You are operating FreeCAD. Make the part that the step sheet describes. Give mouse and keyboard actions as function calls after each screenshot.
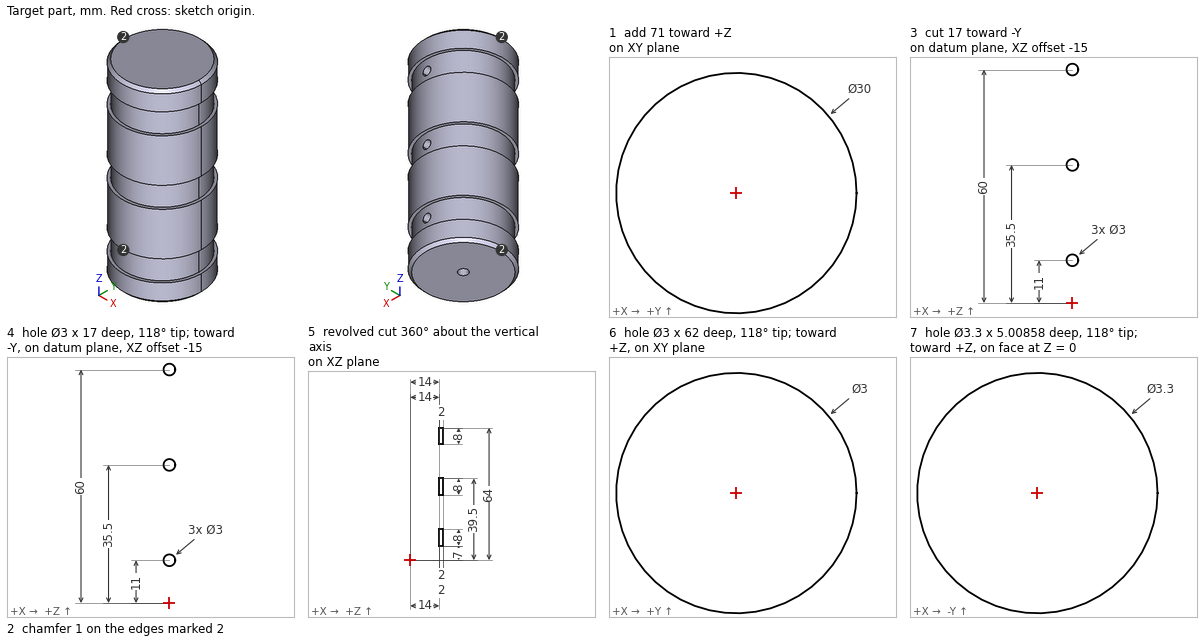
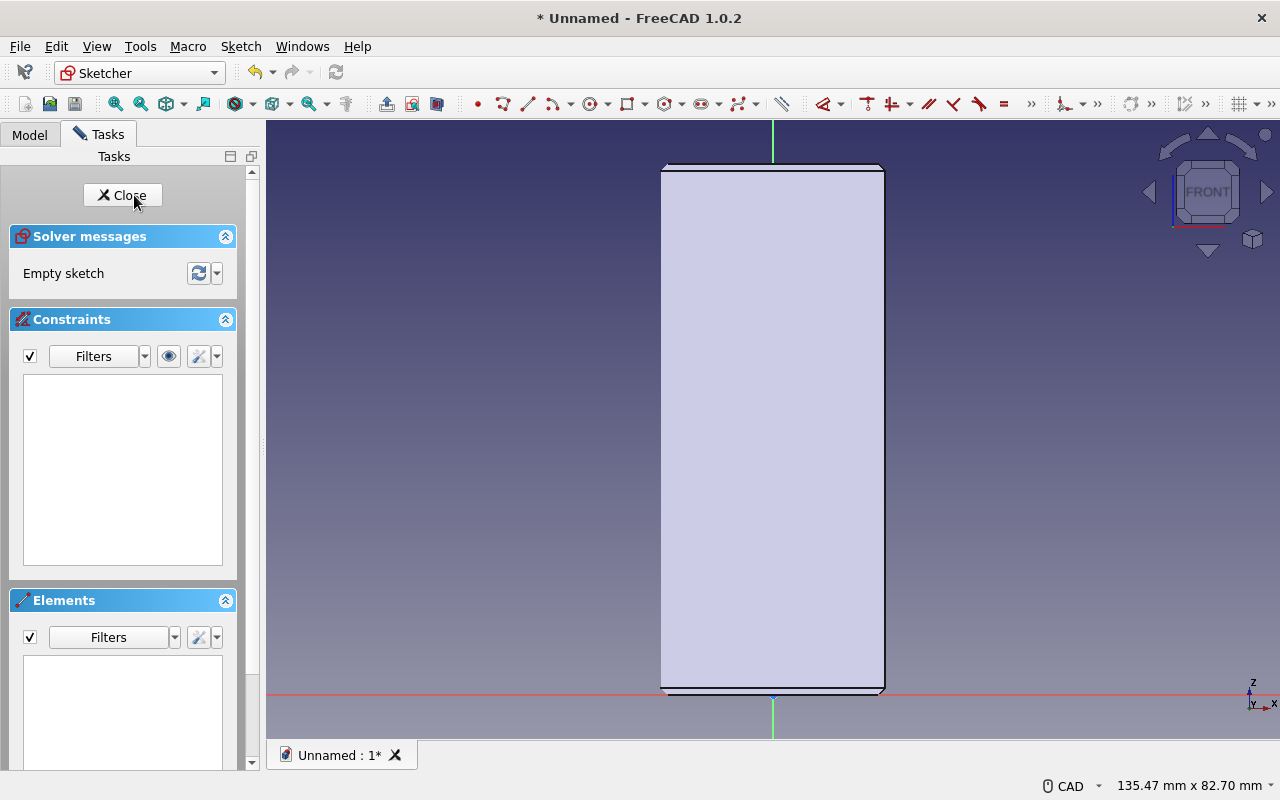
click(437, 104)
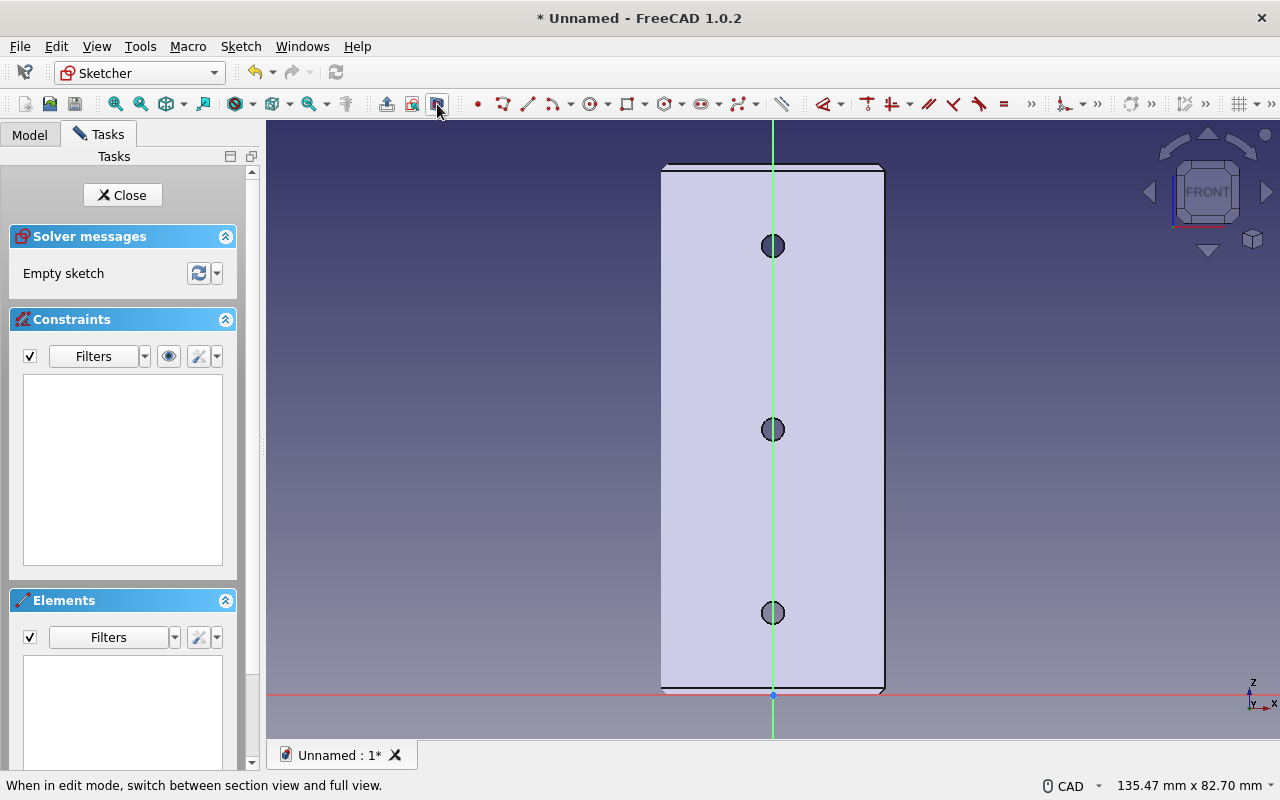
scroll(294, 311, down, 1)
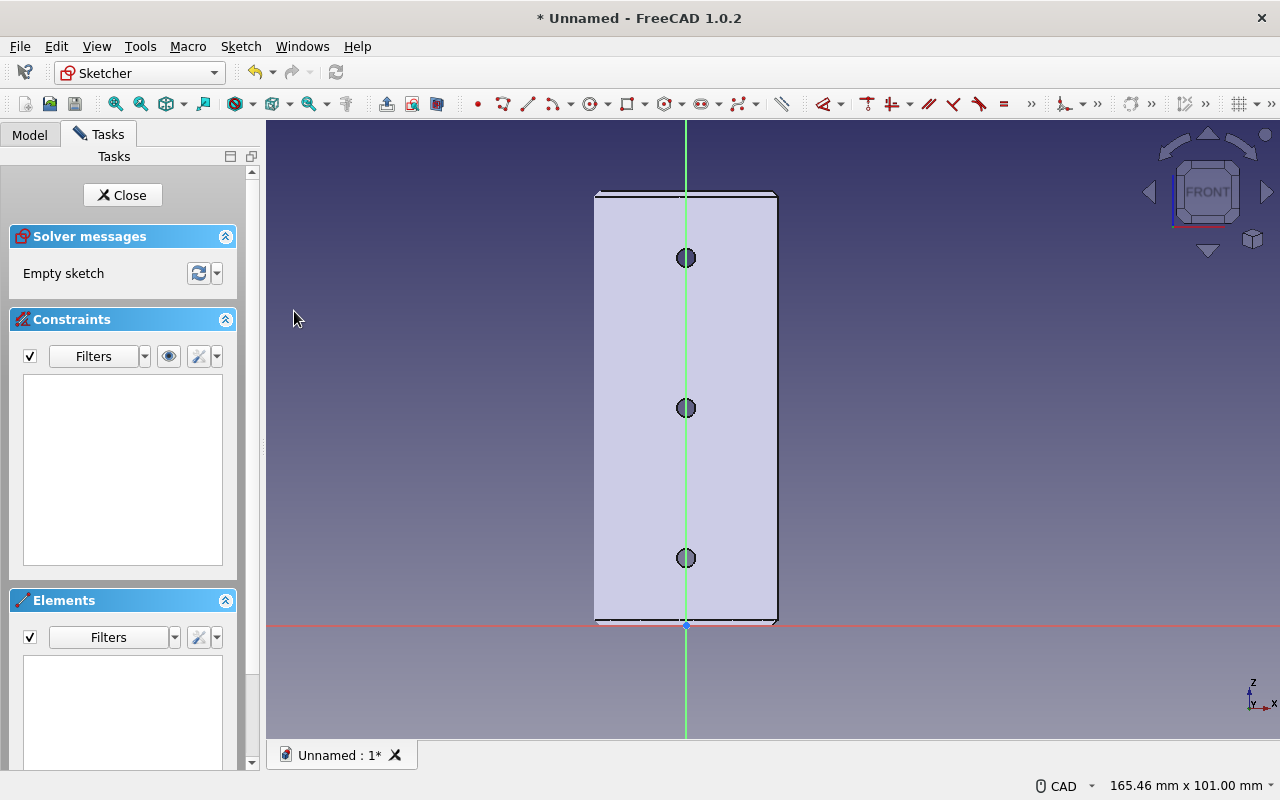
click(626, 104)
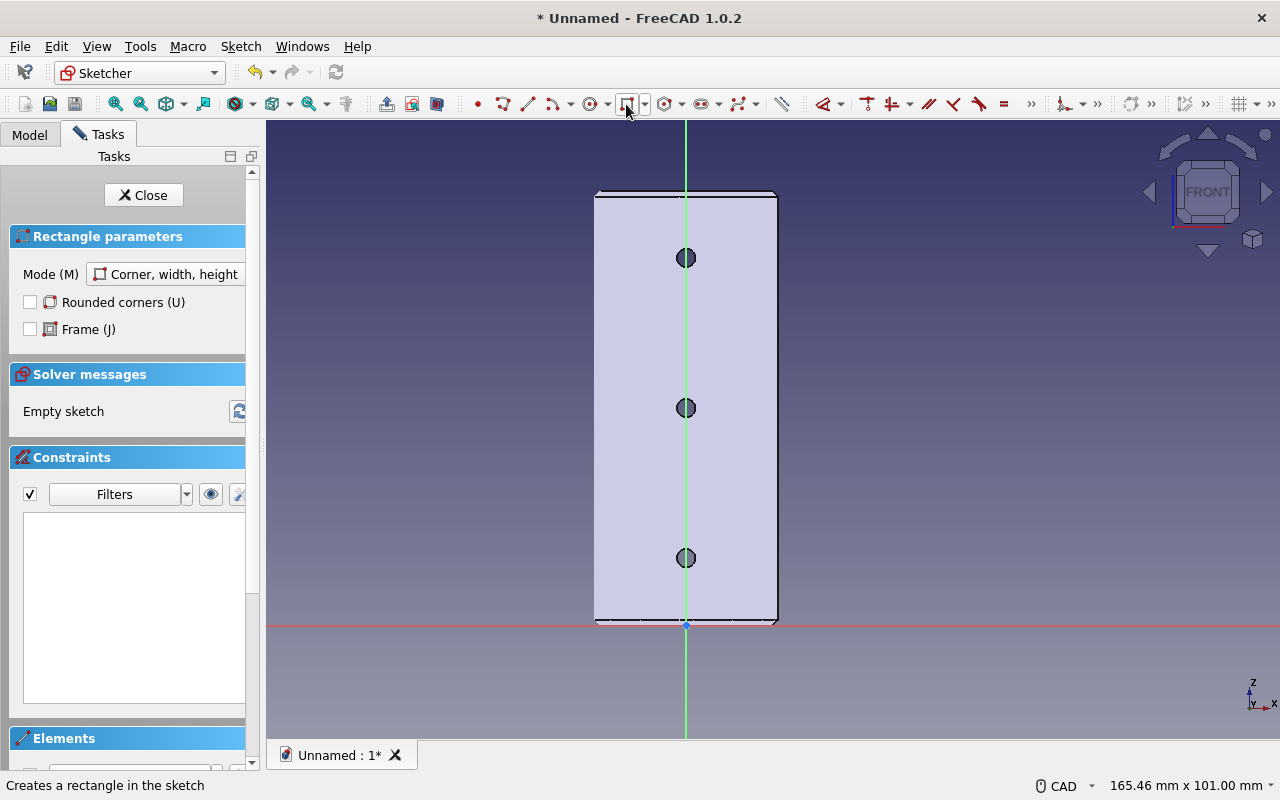
scroll(772, 534, up, 2)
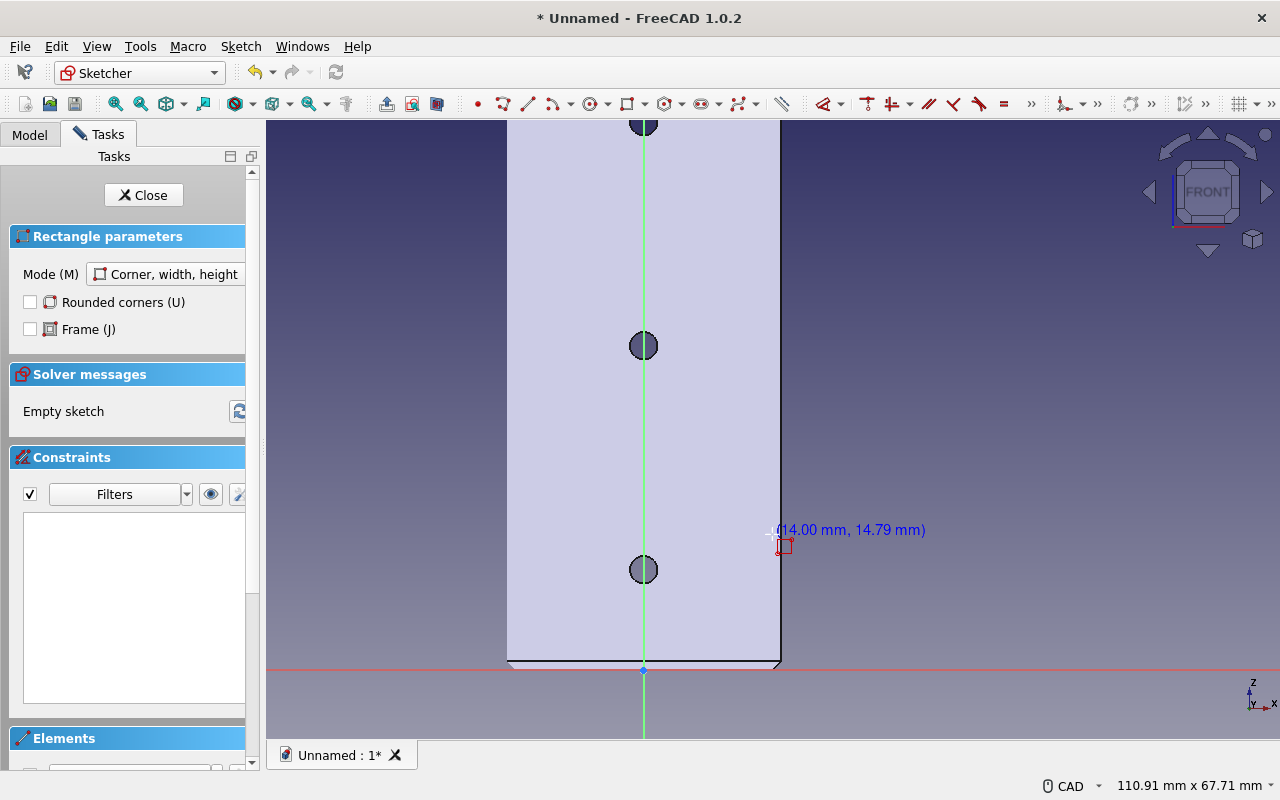
click(772, 533)
move(790, 606)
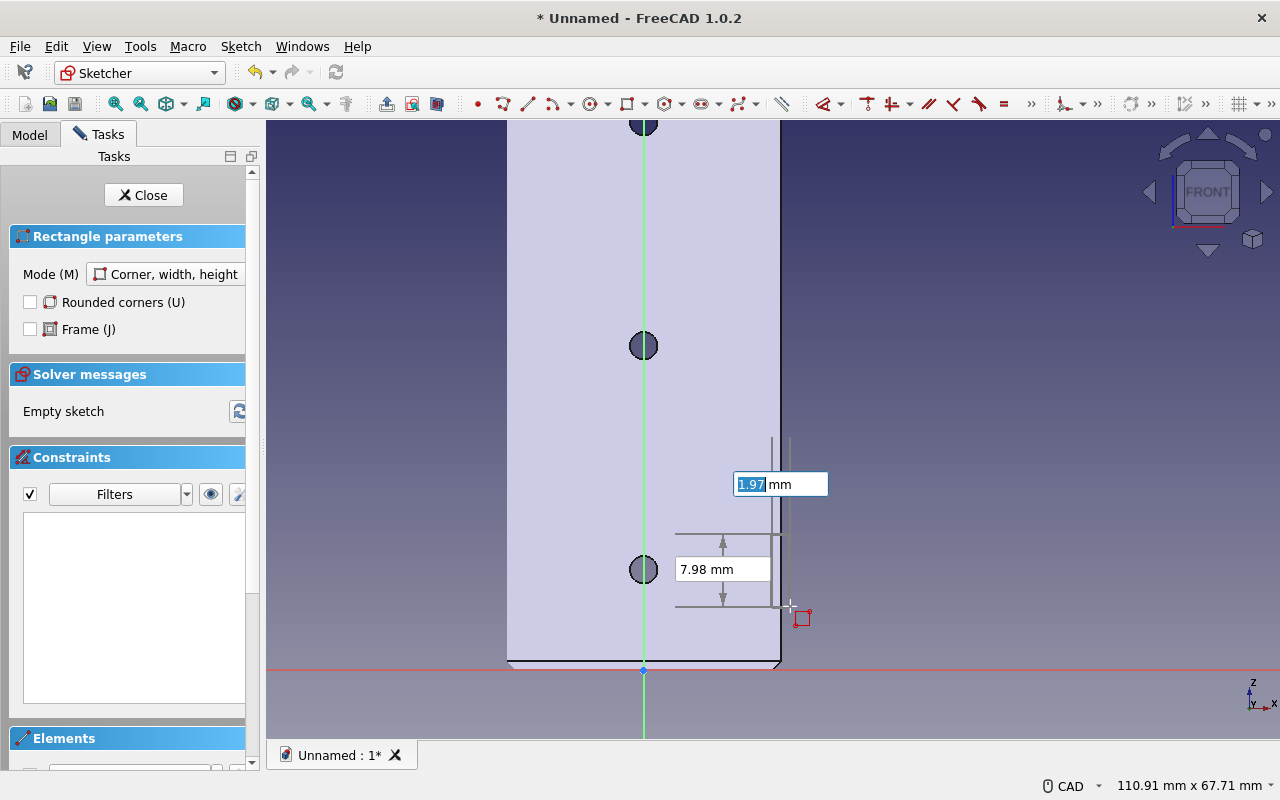
text(2)
key(Tab)
text(8)
key(Return)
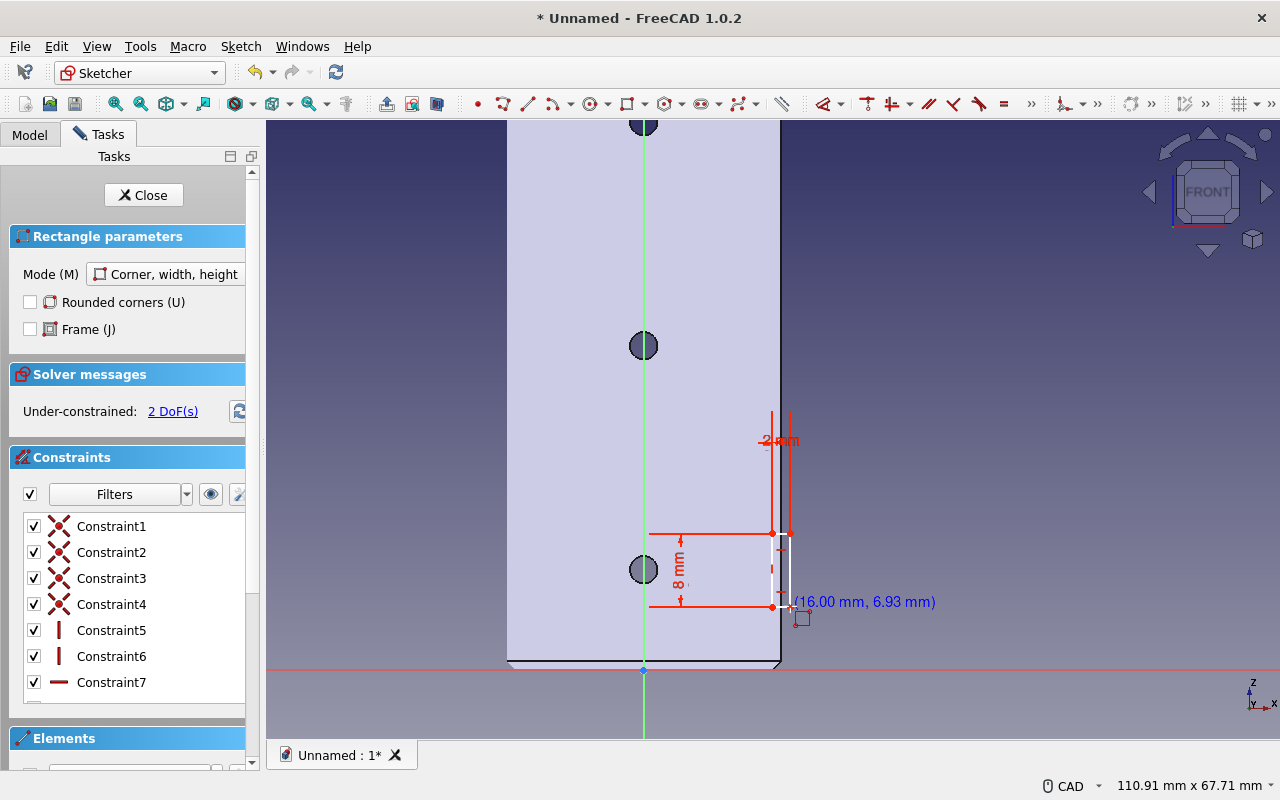
click(772, 309)
move(790, 382)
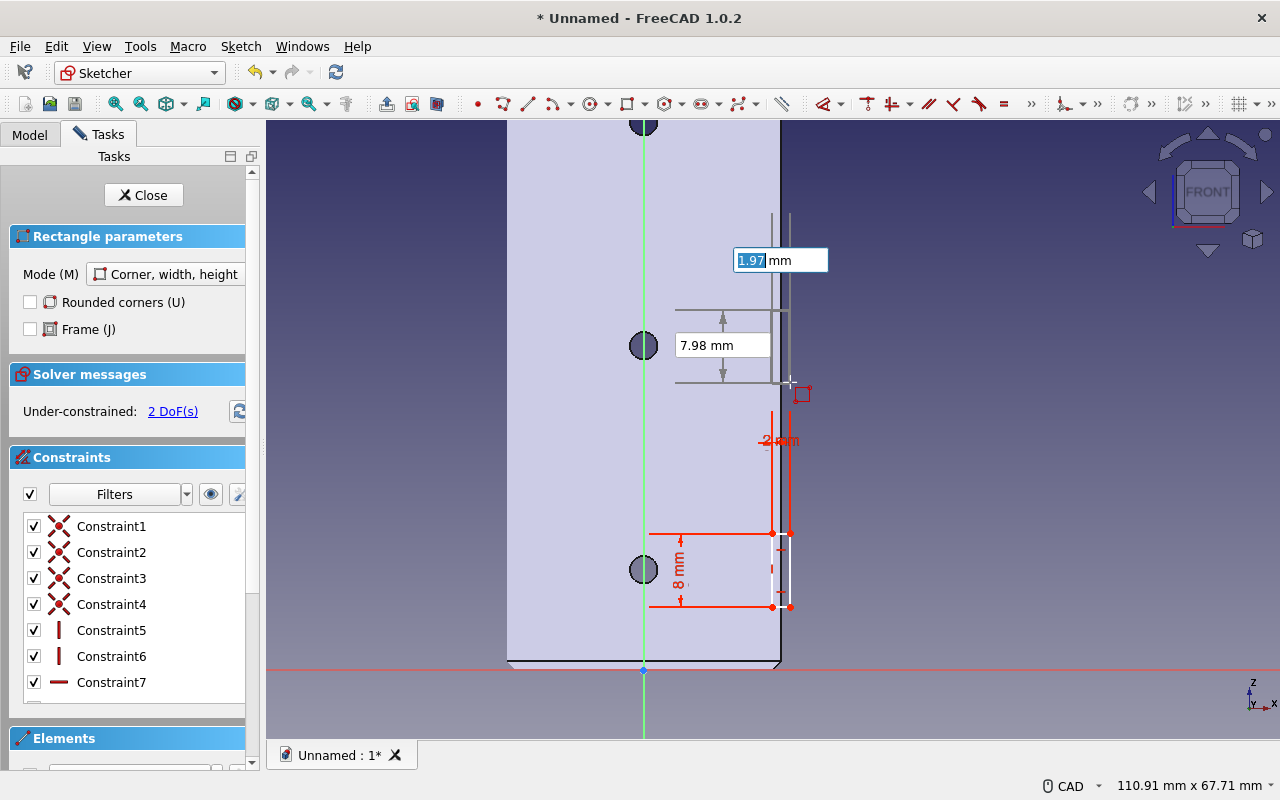
text(2)
key(Tab)
text(8)
key(Return)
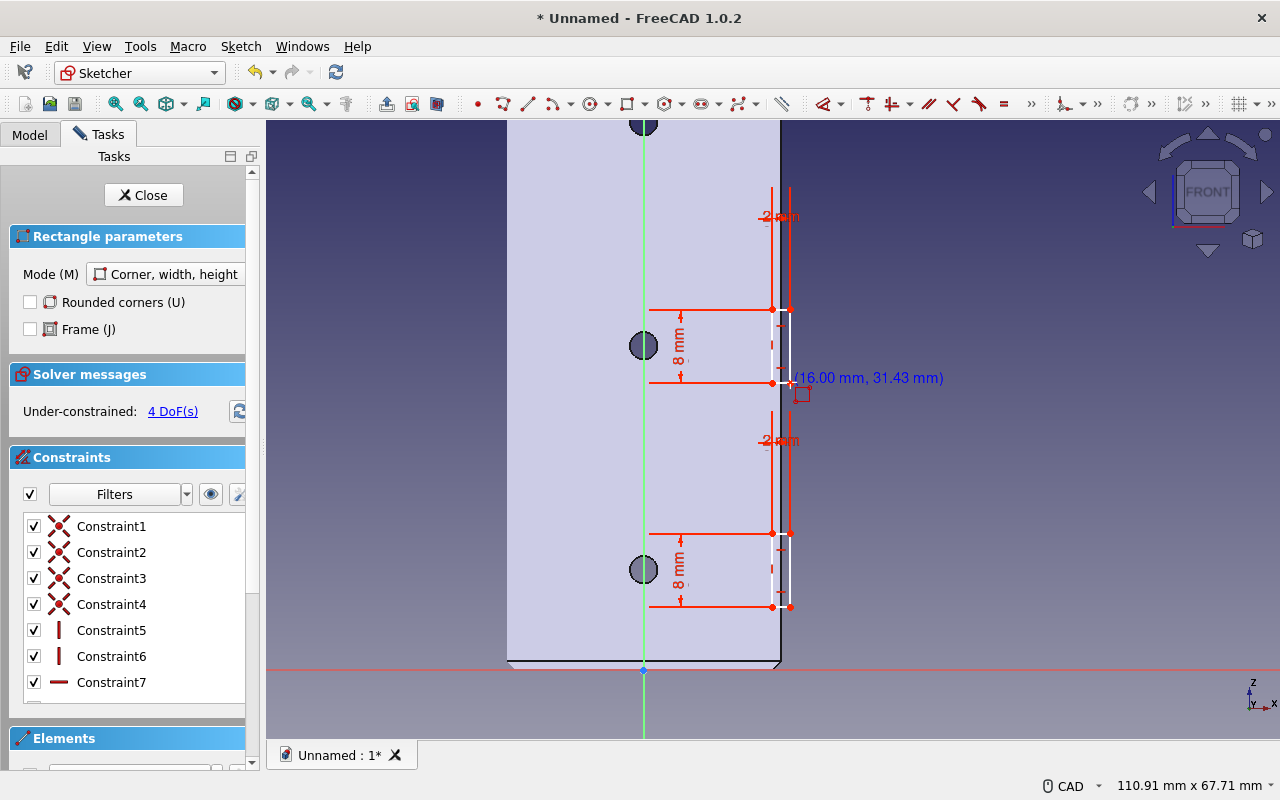
scroll(679, 535, down, 2)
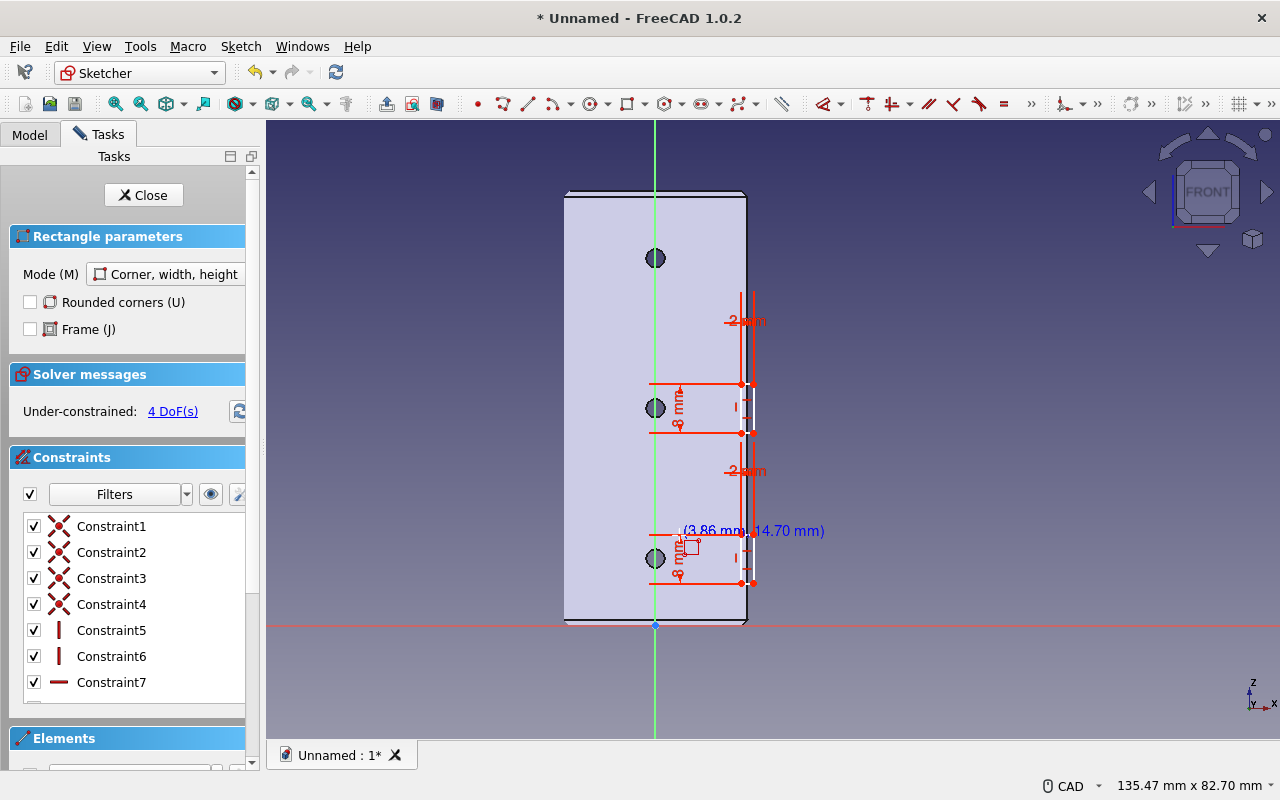
scroll(741, 234, up, 2)